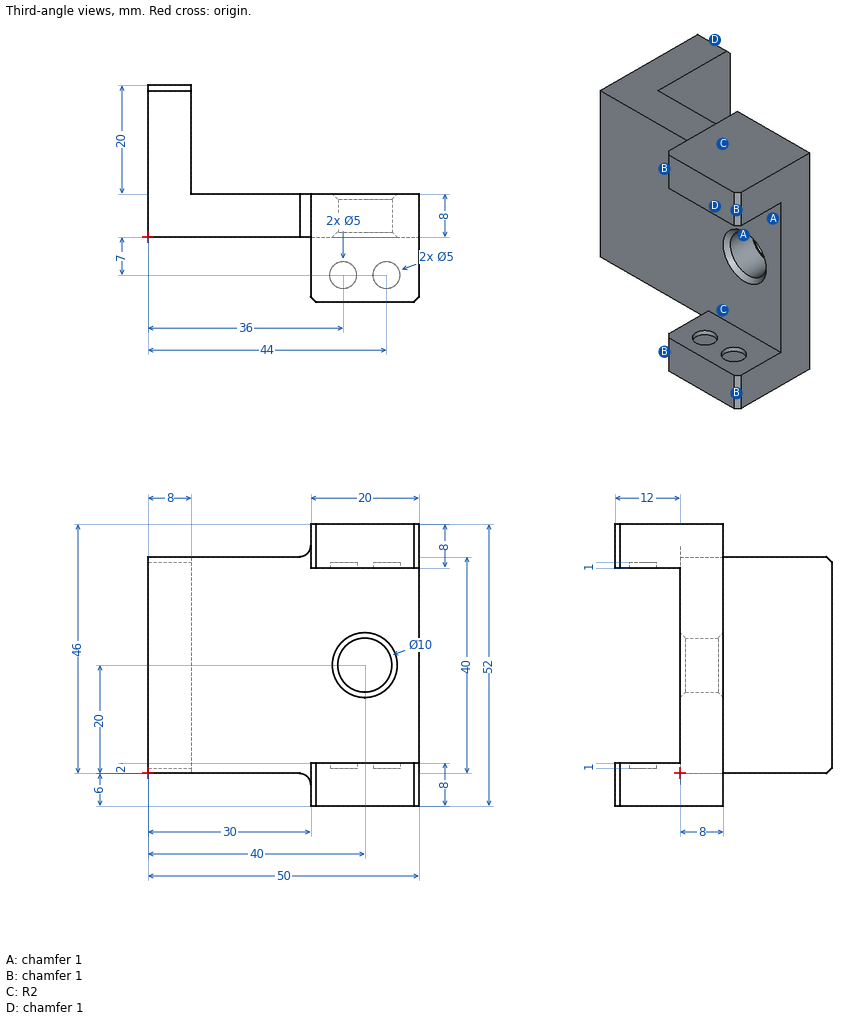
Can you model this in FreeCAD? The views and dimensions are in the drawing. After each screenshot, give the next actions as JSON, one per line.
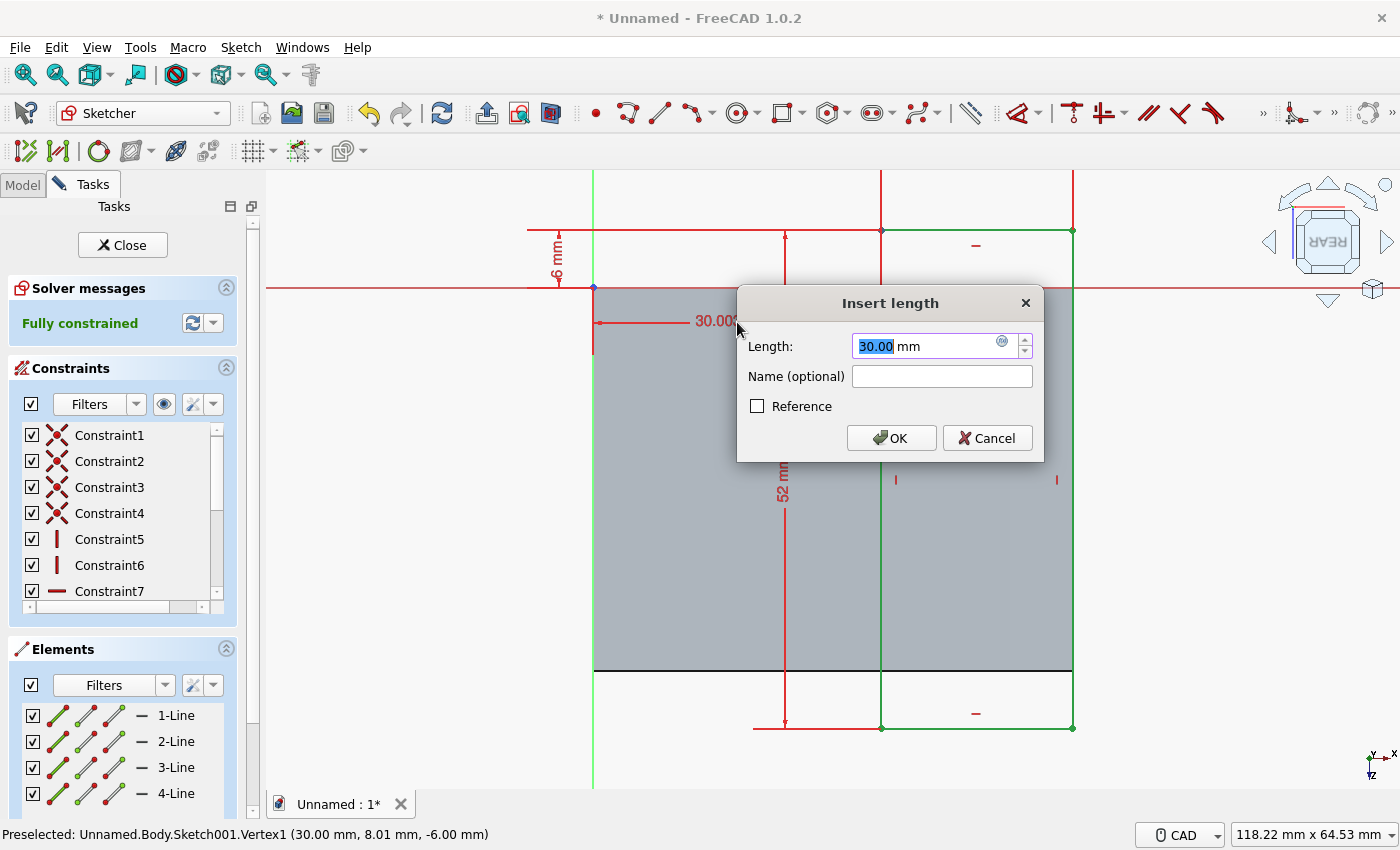
{"action": "type", "text": "30"}
{"action": "key", "text": "Return"}
{"action": "key", "text": "Escape"}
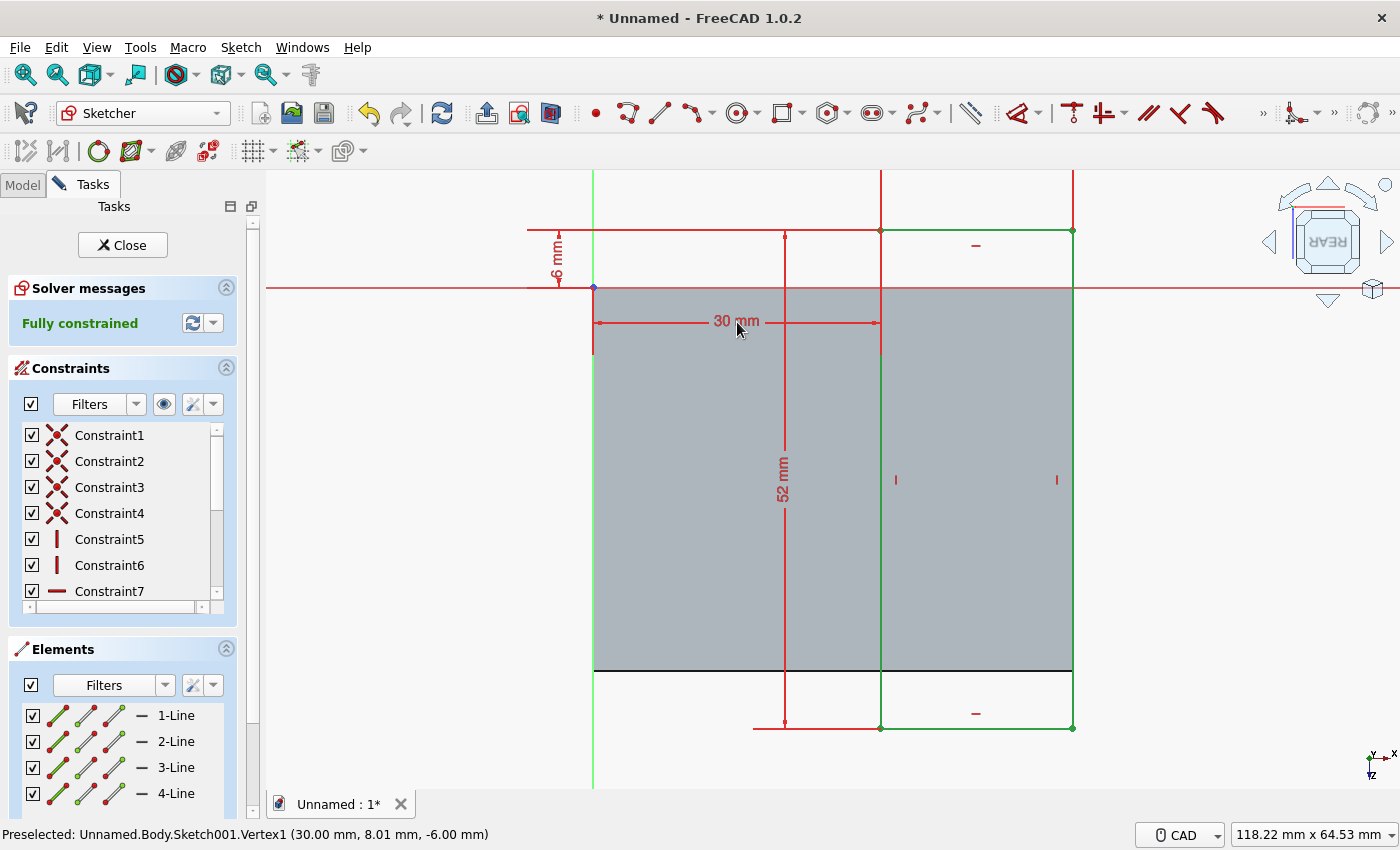
{"action": "left_click", "coordinate": [123, 245]}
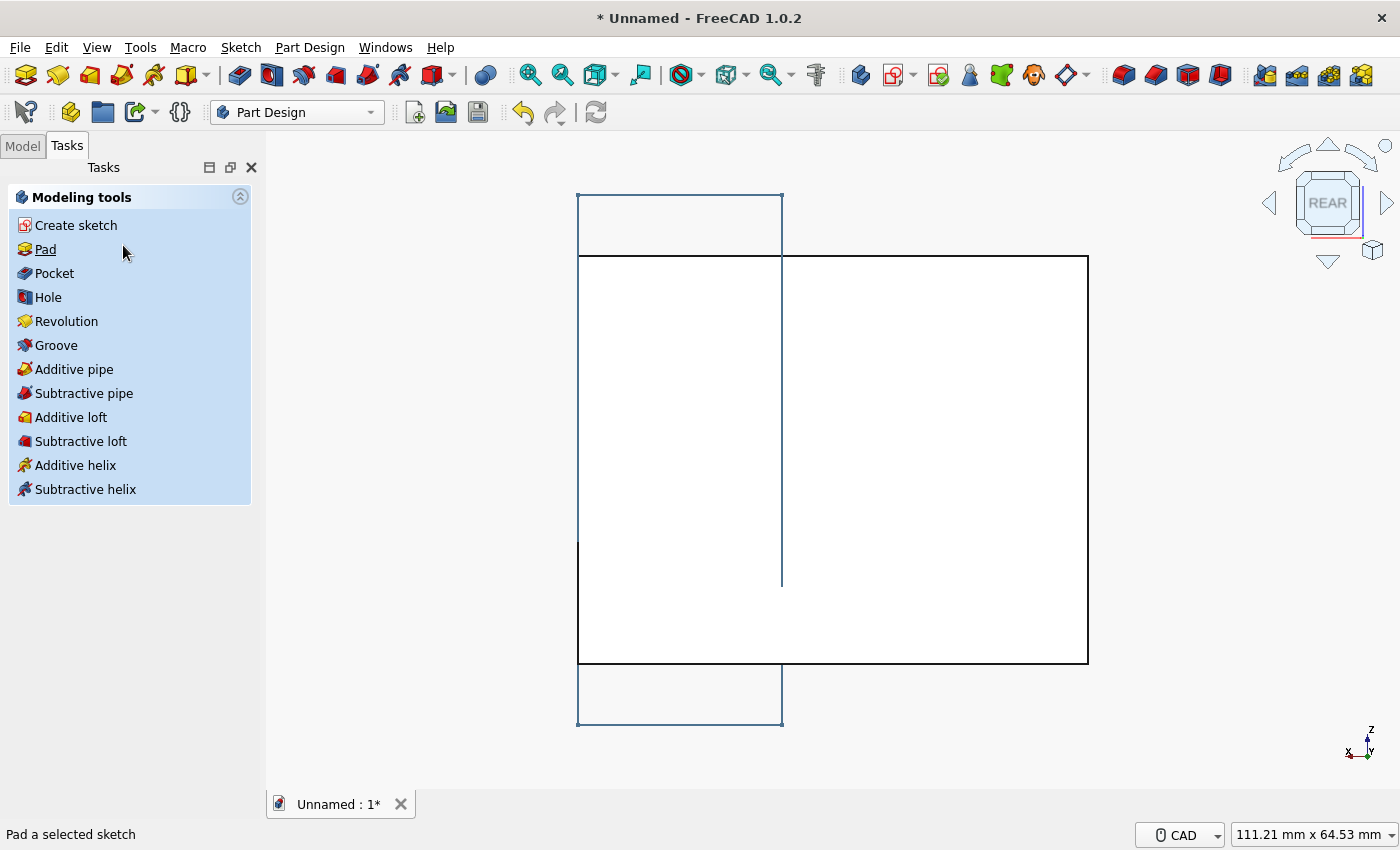
{"action": "left_click", "coordinate": [26, 76]}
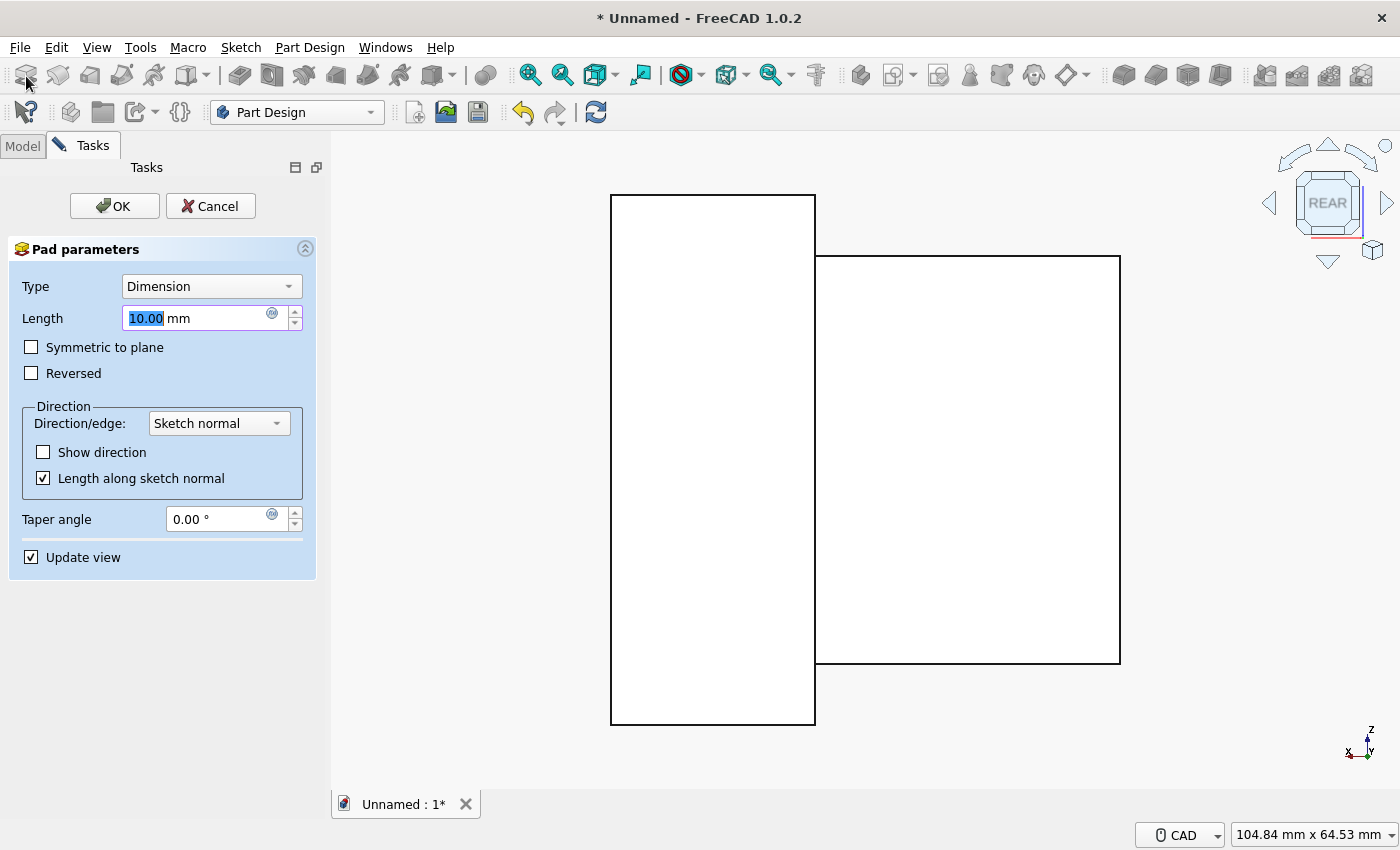
{"action": "type", "text": "8"}
{"action": "key", "text": "Tab"}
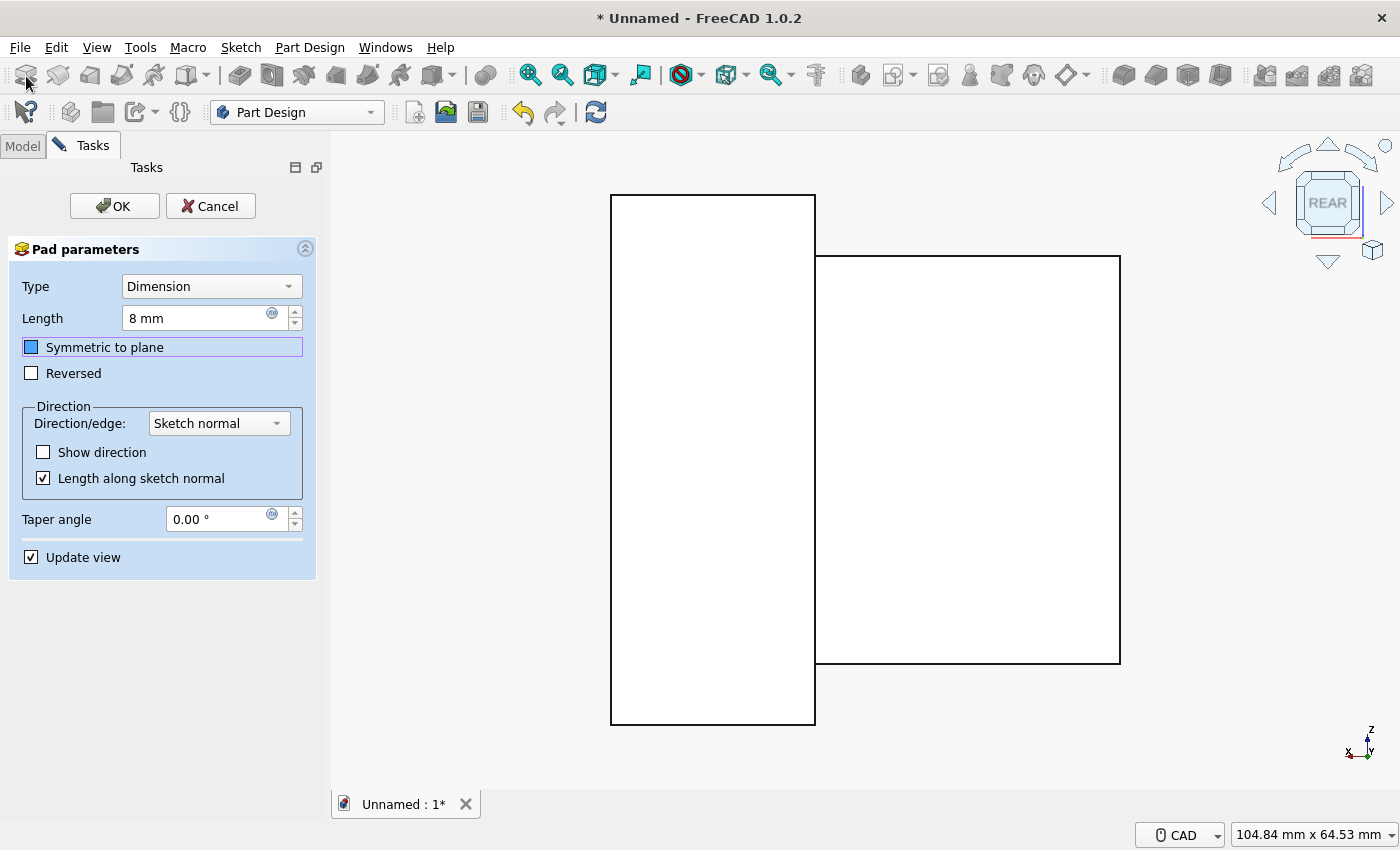
{"action": "left_click", "coordinate": [30, 373]}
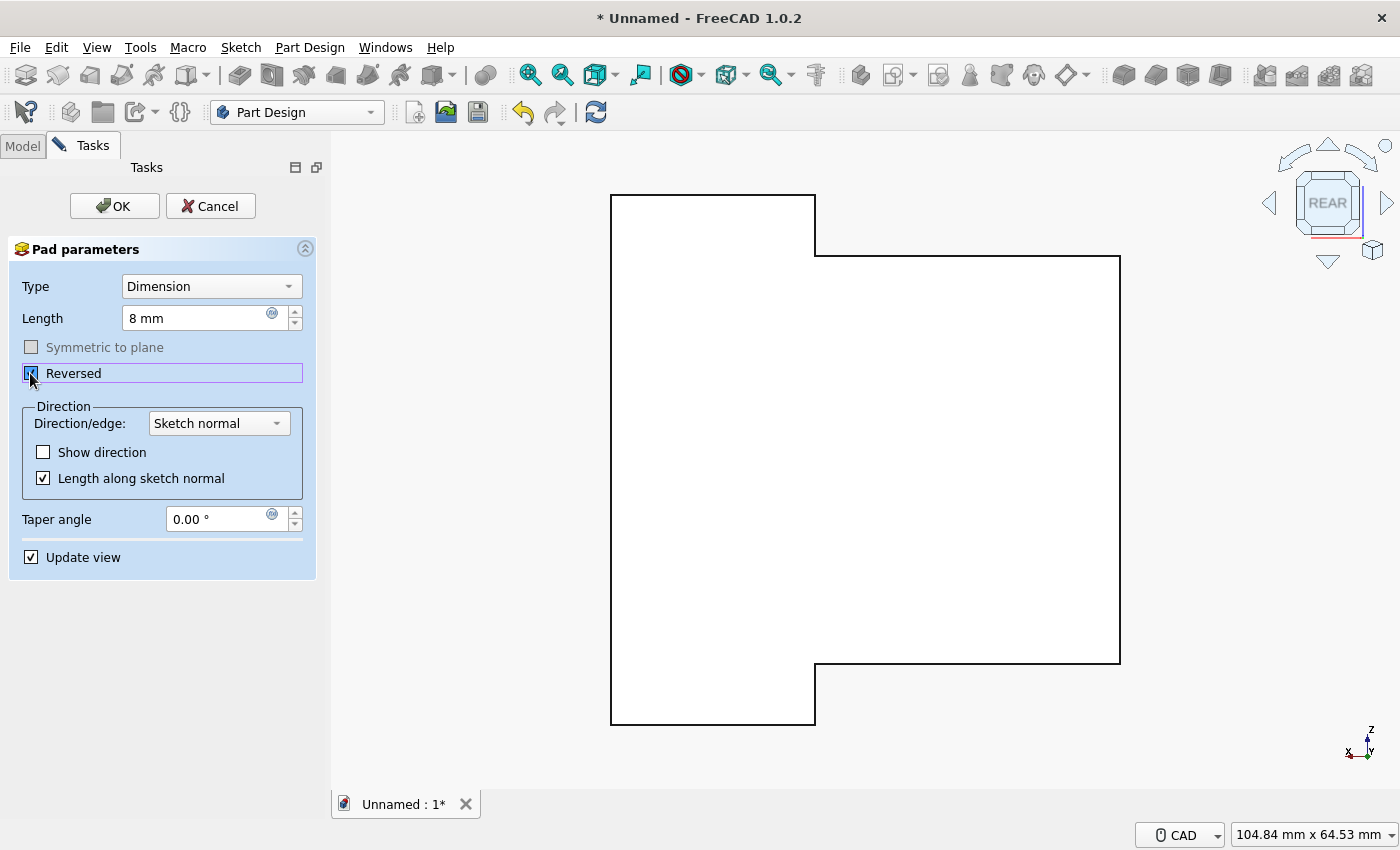
{"action": "left_click", "coordinate": [115, 206]}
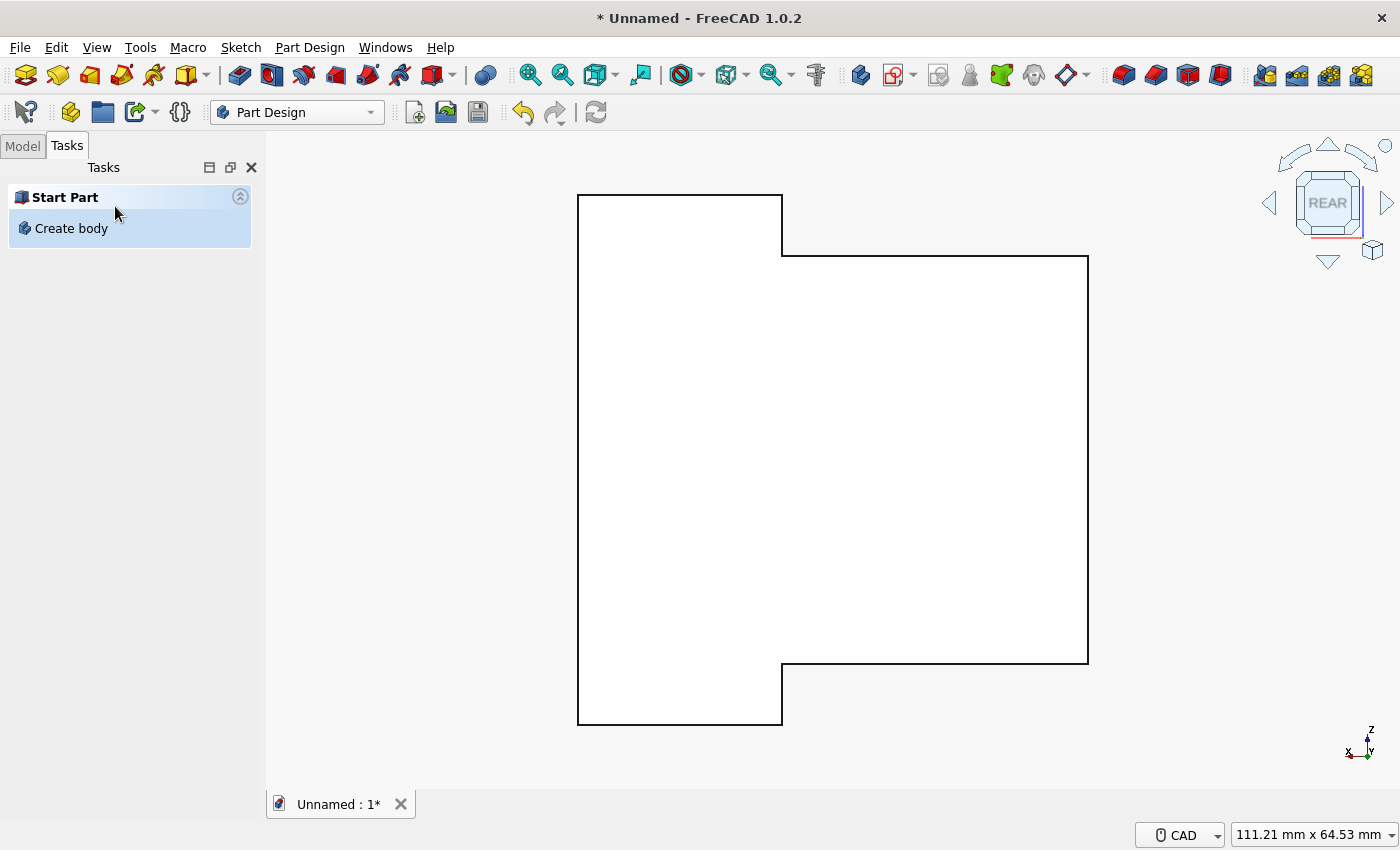
{"action": "key", "text": "0"}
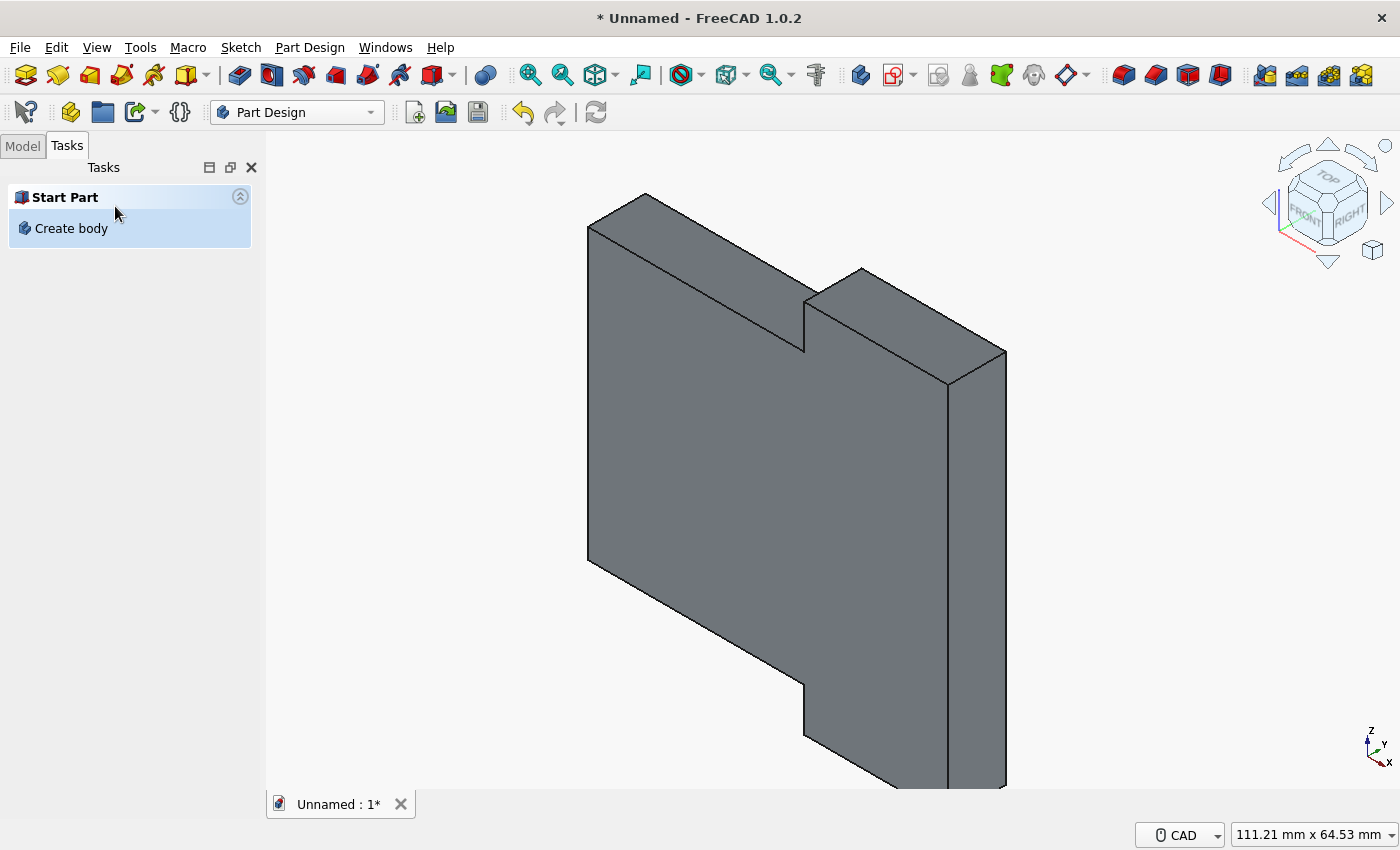
{"action": "left_click", "coordinate": [532, 76]}